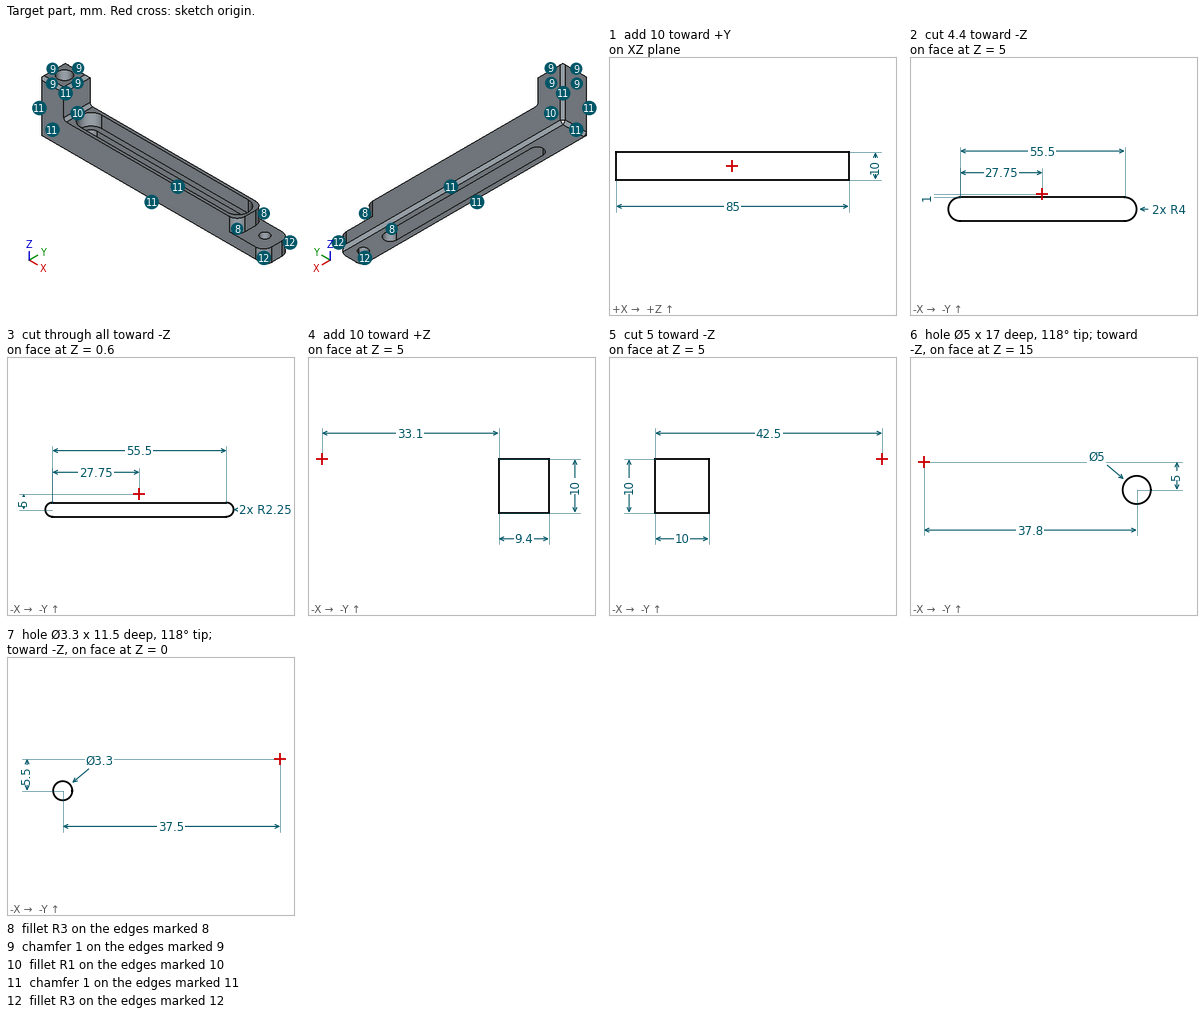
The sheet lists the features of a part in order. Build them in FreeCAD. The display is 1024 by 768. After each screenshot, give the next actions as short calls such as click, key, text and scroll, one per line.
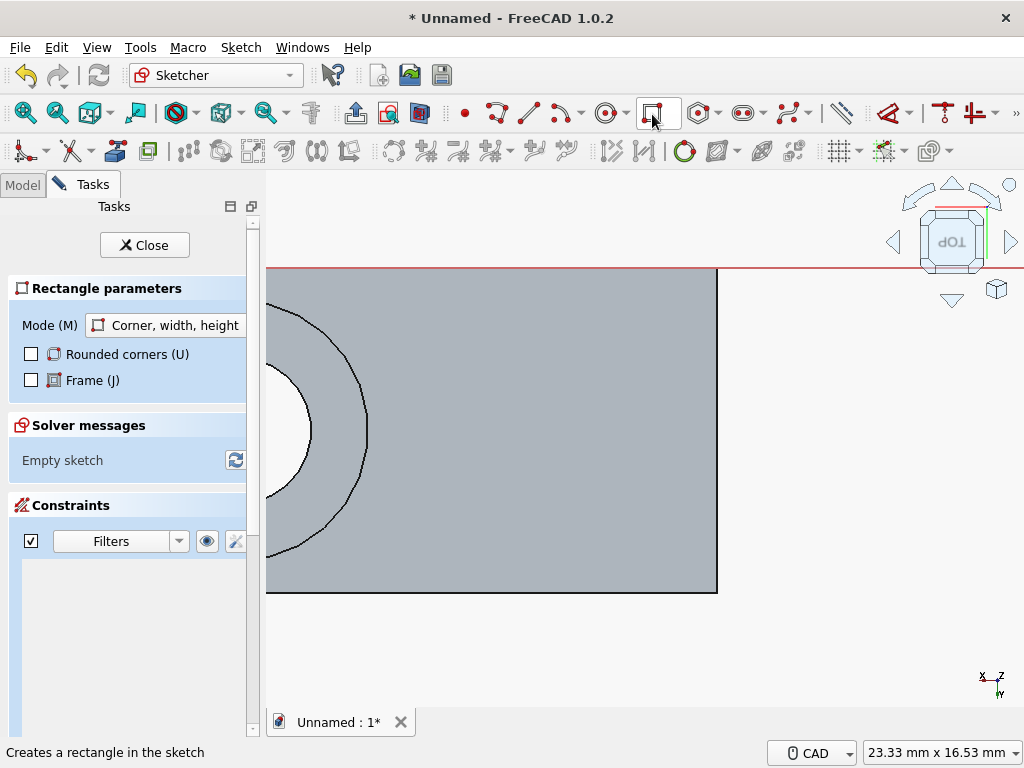
click(412, 268)
click(717, 593)
key(Escape)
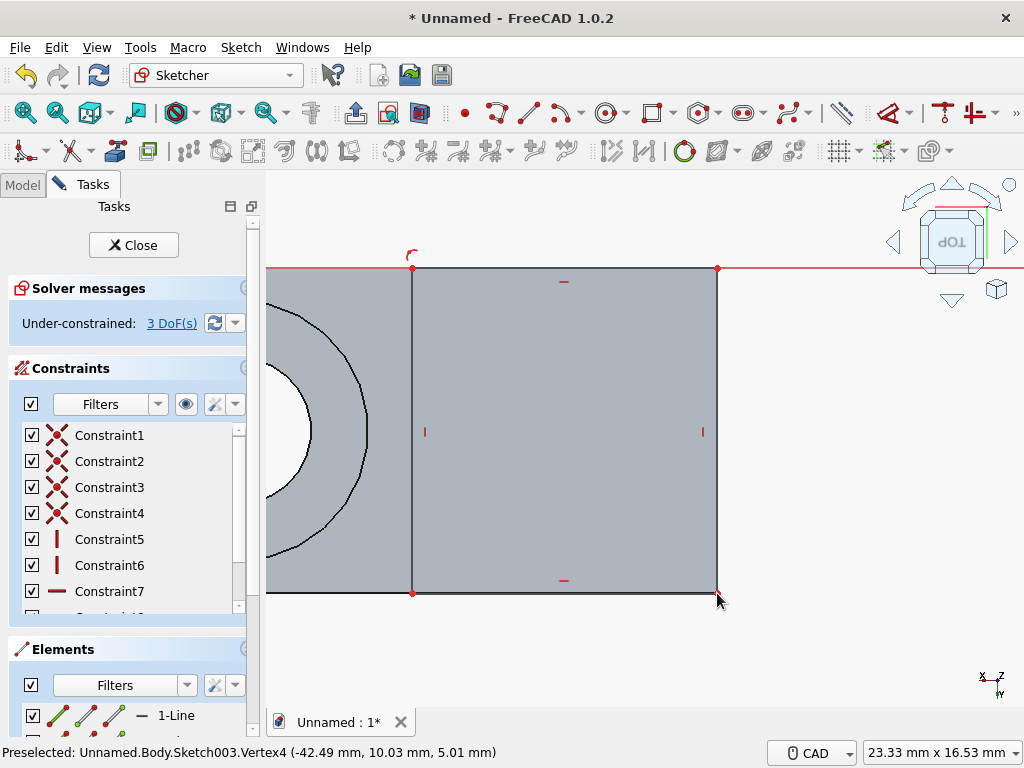
key(d)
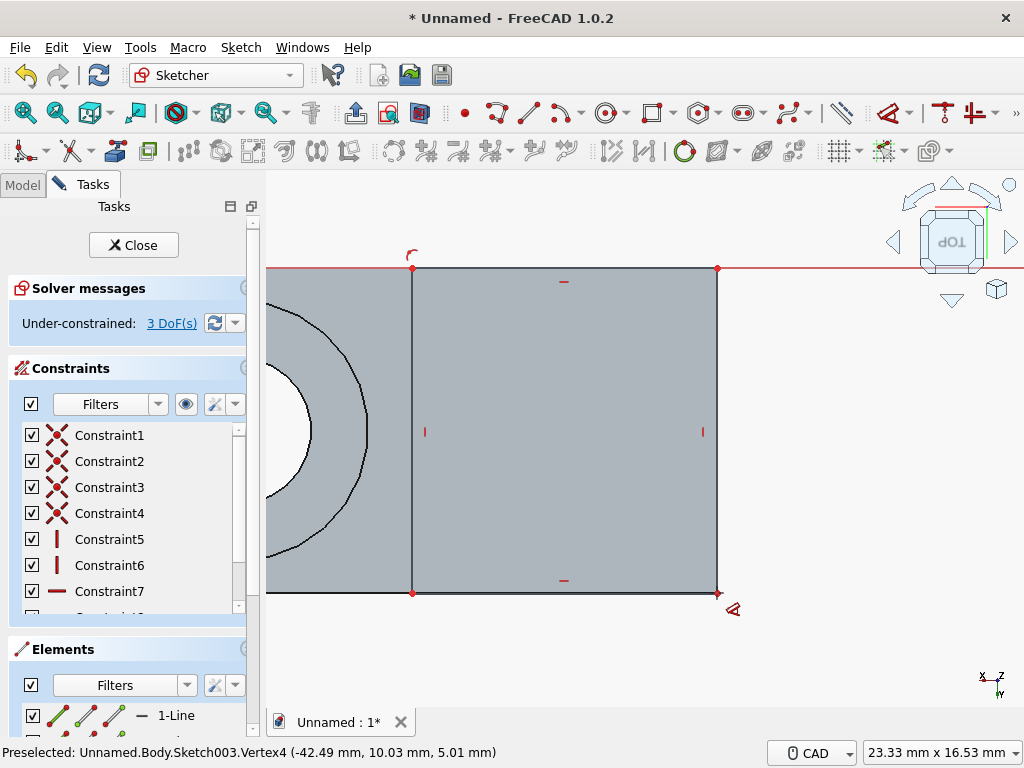
click(412, 366)
click(378, 431)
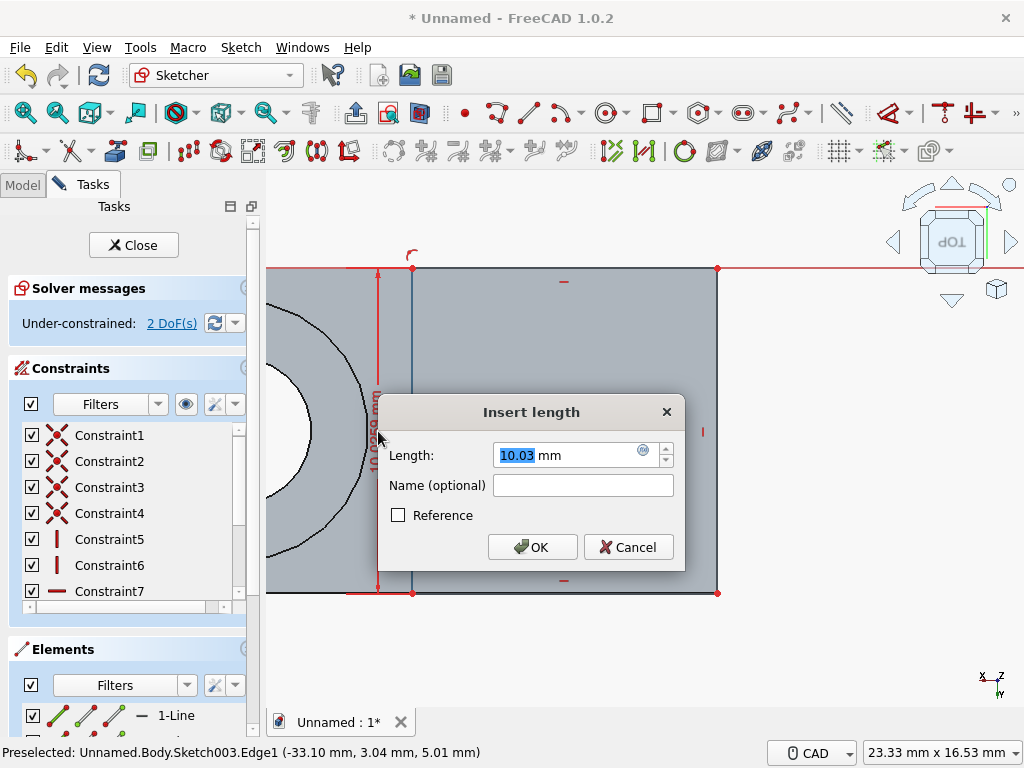
text(10)
key(Return)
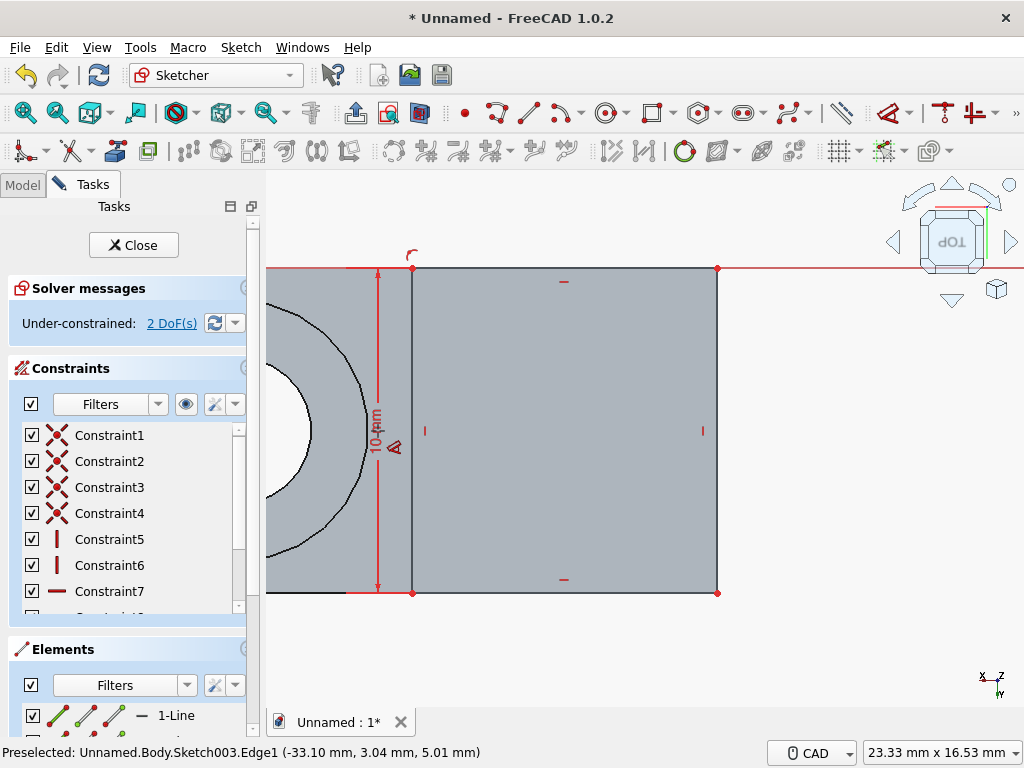
click(503, 593)
click(564, 627)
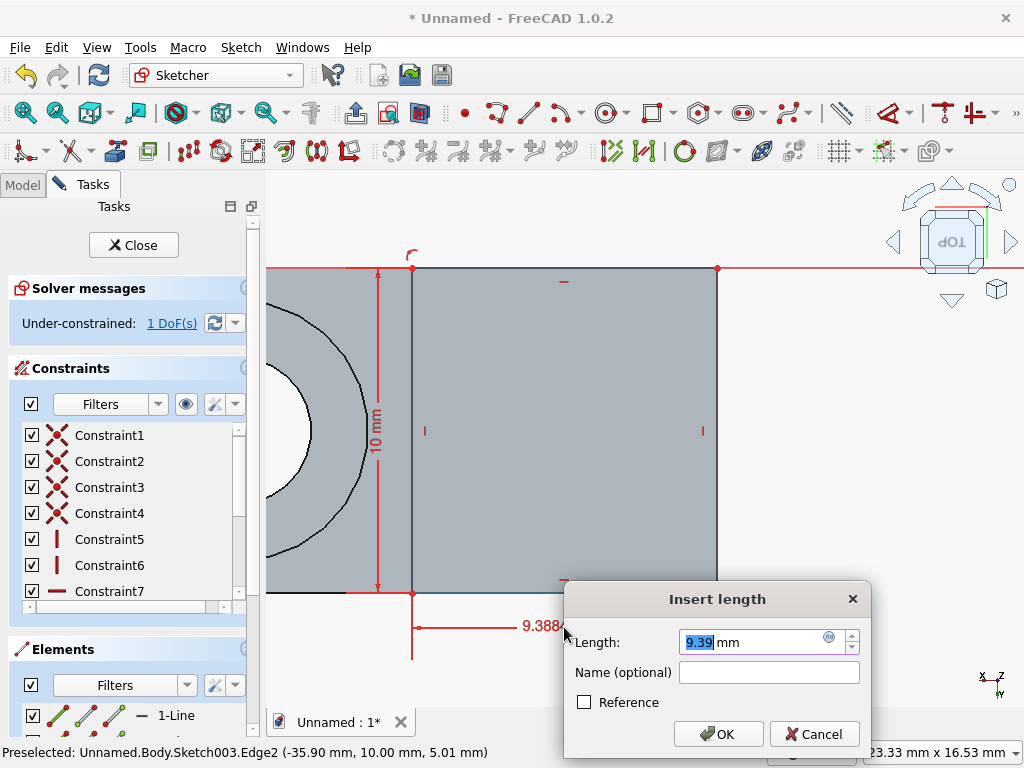
text(9.4)
key(Return)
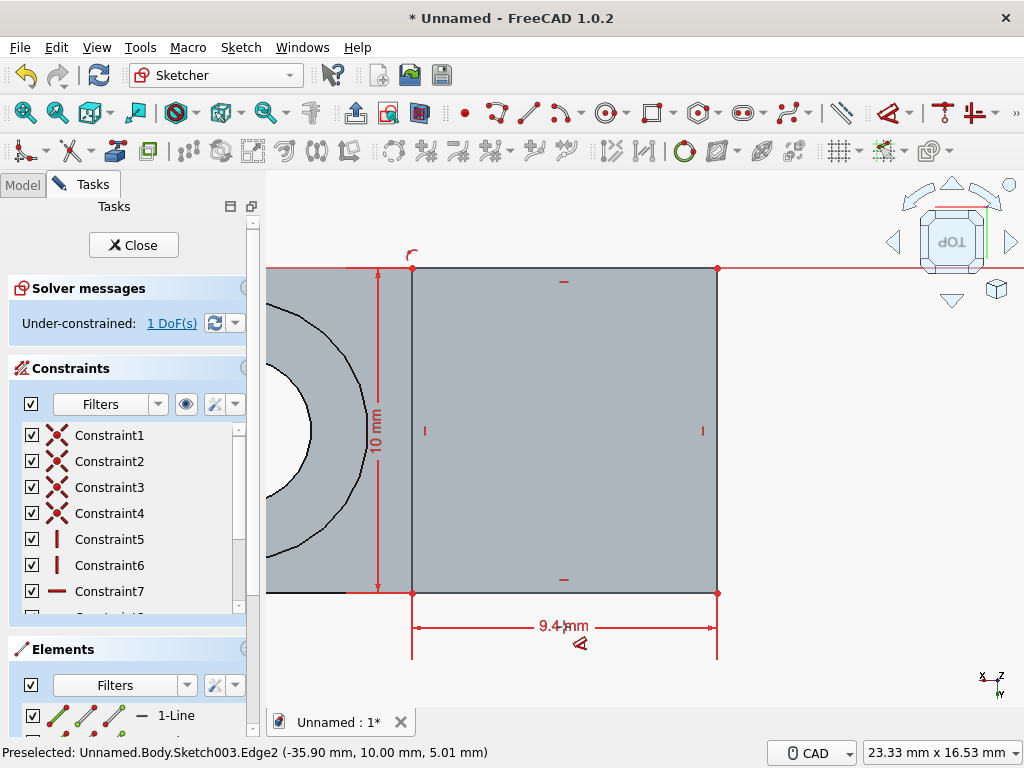
click(412, 268)
click(353, 234)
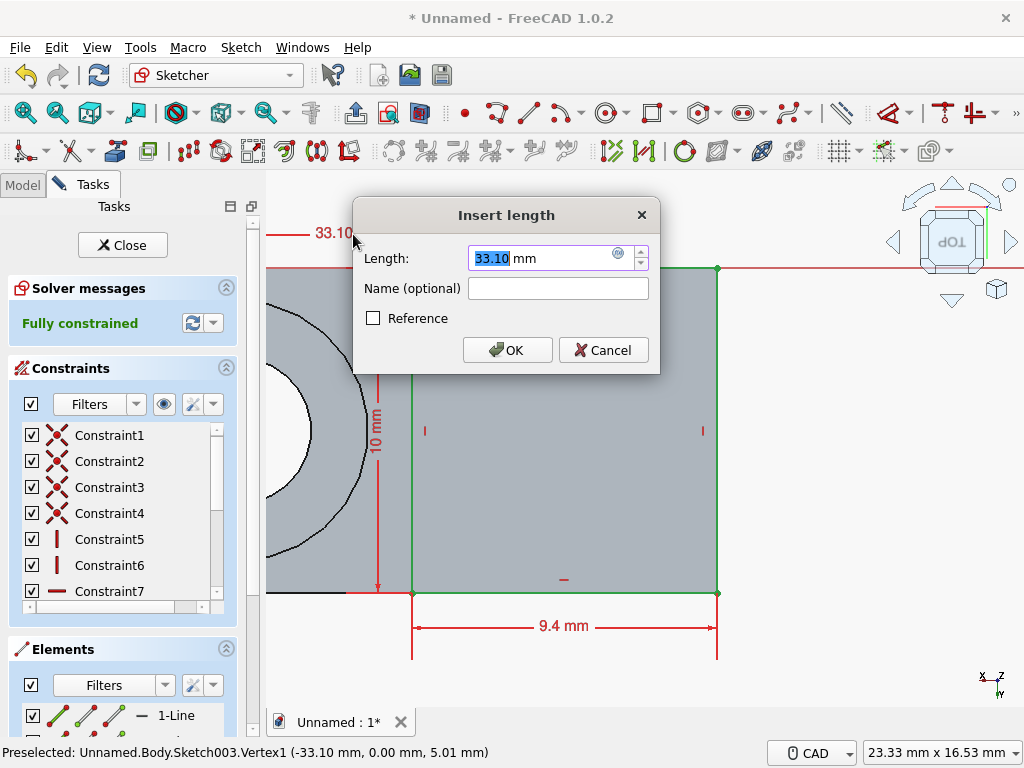
text(33.1)
key(Return)
key(Escape)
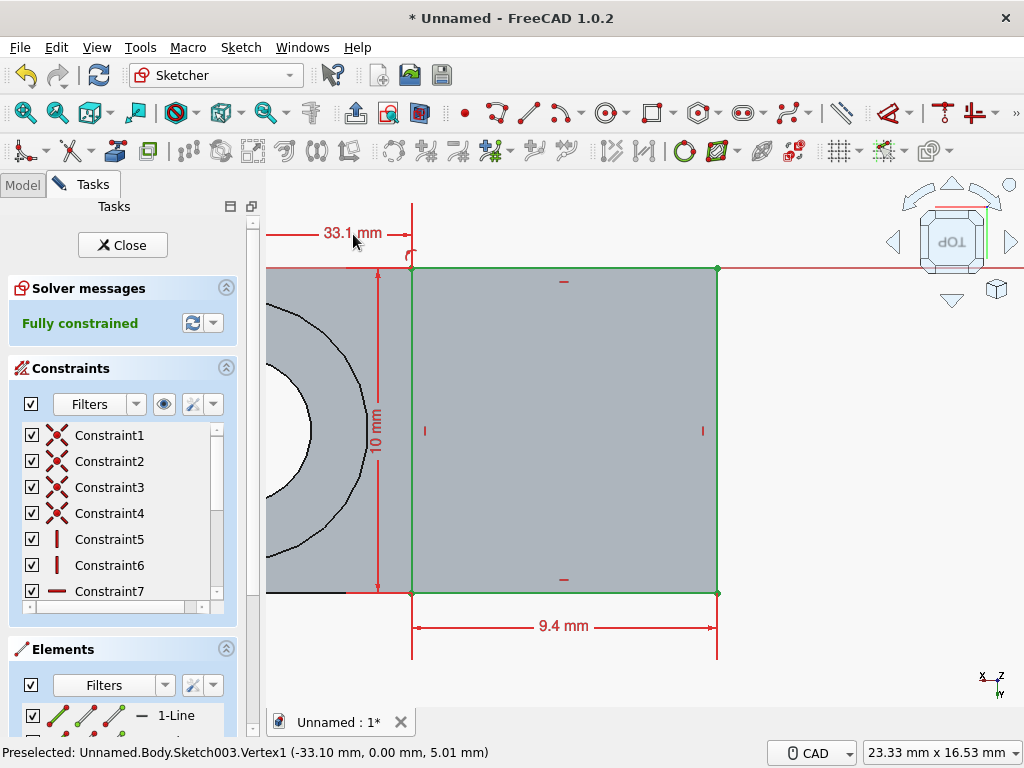
click(123, 245)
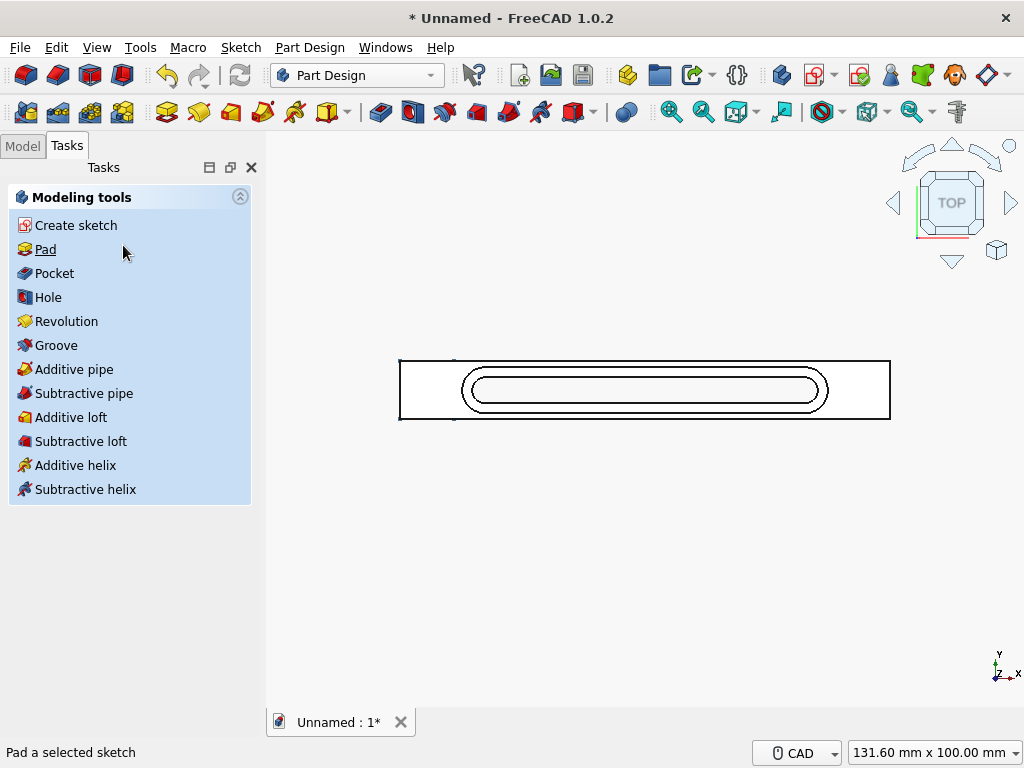
click(168, 112)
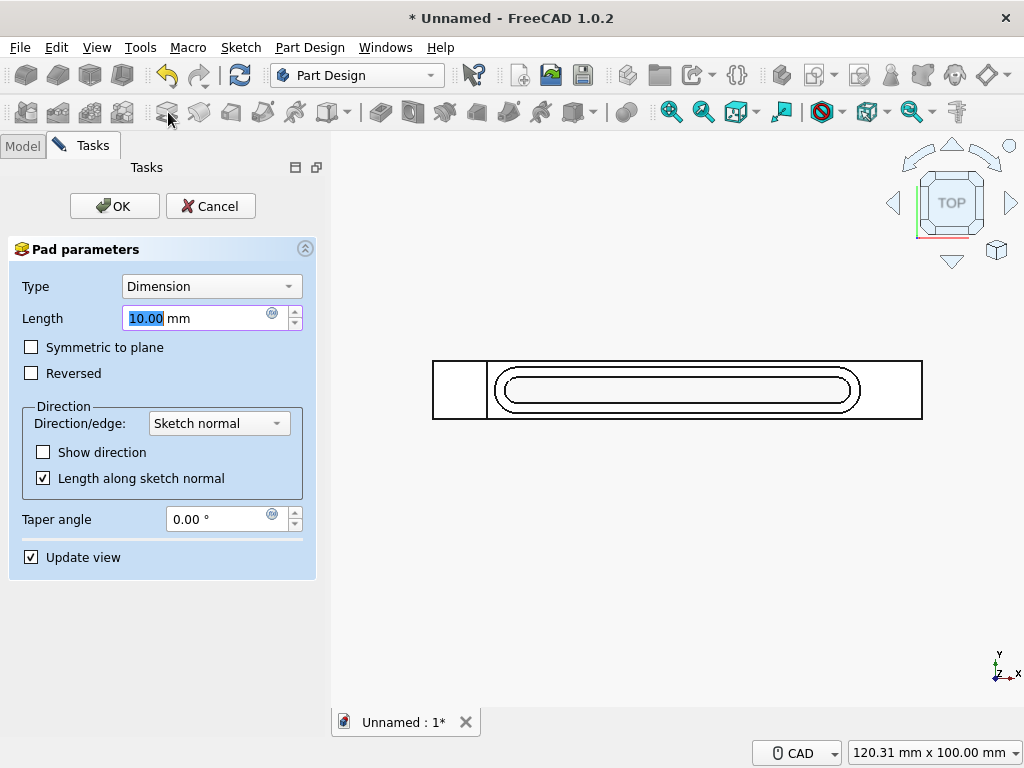
text(10)
key(Tab)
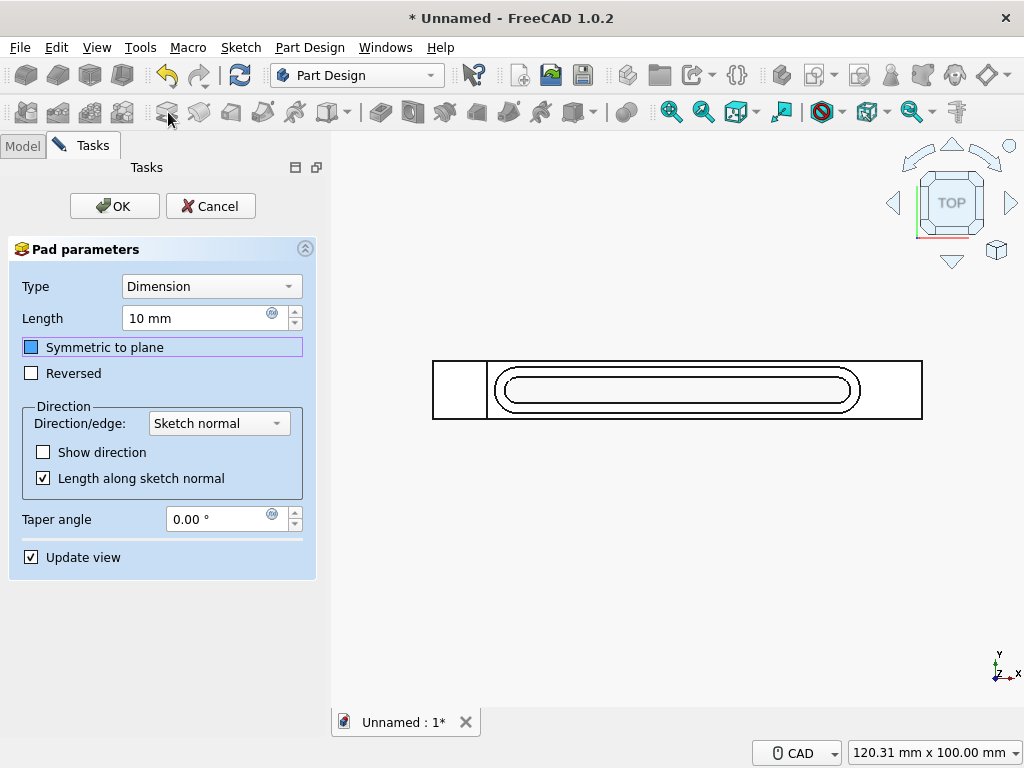
click(115, 206)